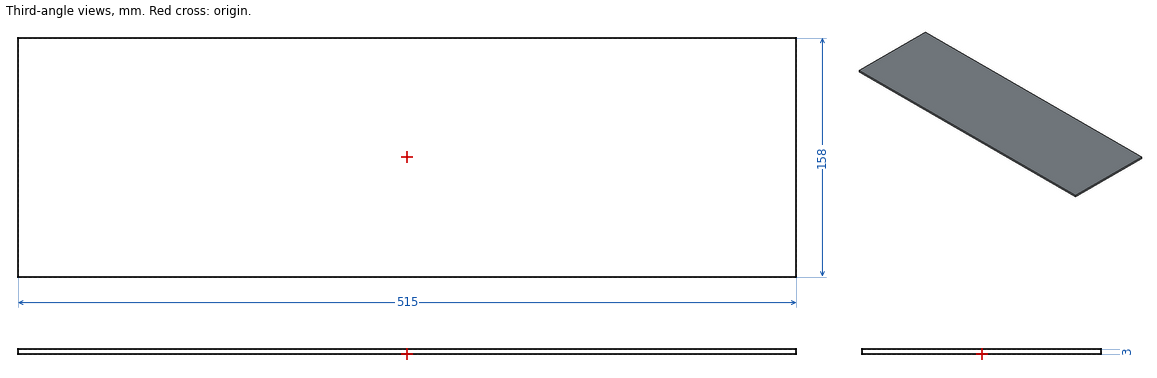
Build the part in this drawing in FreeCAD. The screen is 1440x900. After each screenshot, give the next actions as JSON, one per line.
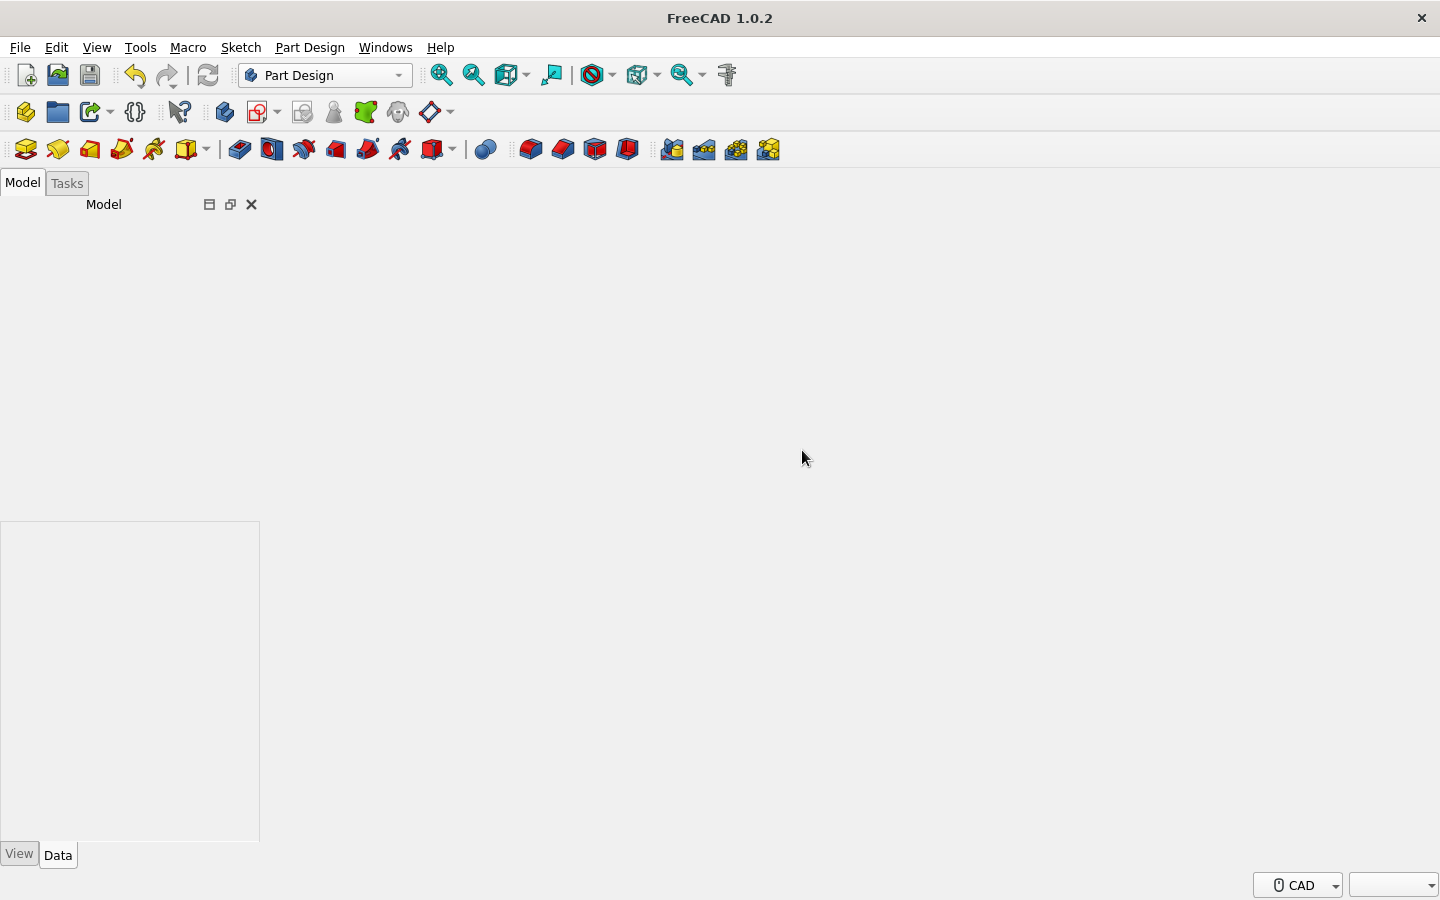
{"action": "left_click", "coordinate": [26, 76]}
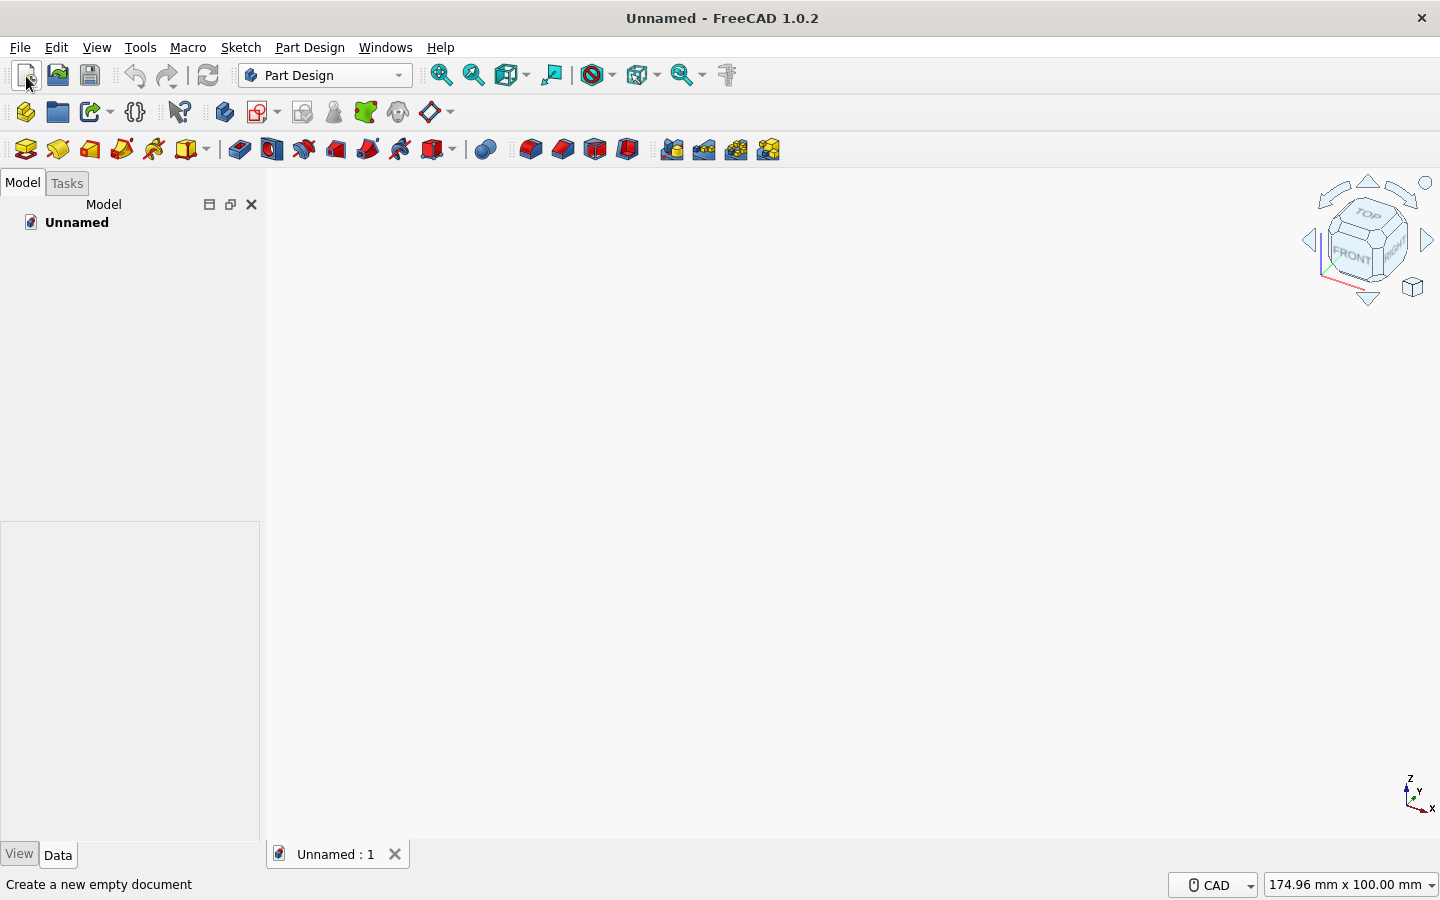
{"action": "left_click", "coordinate": [258, 112]}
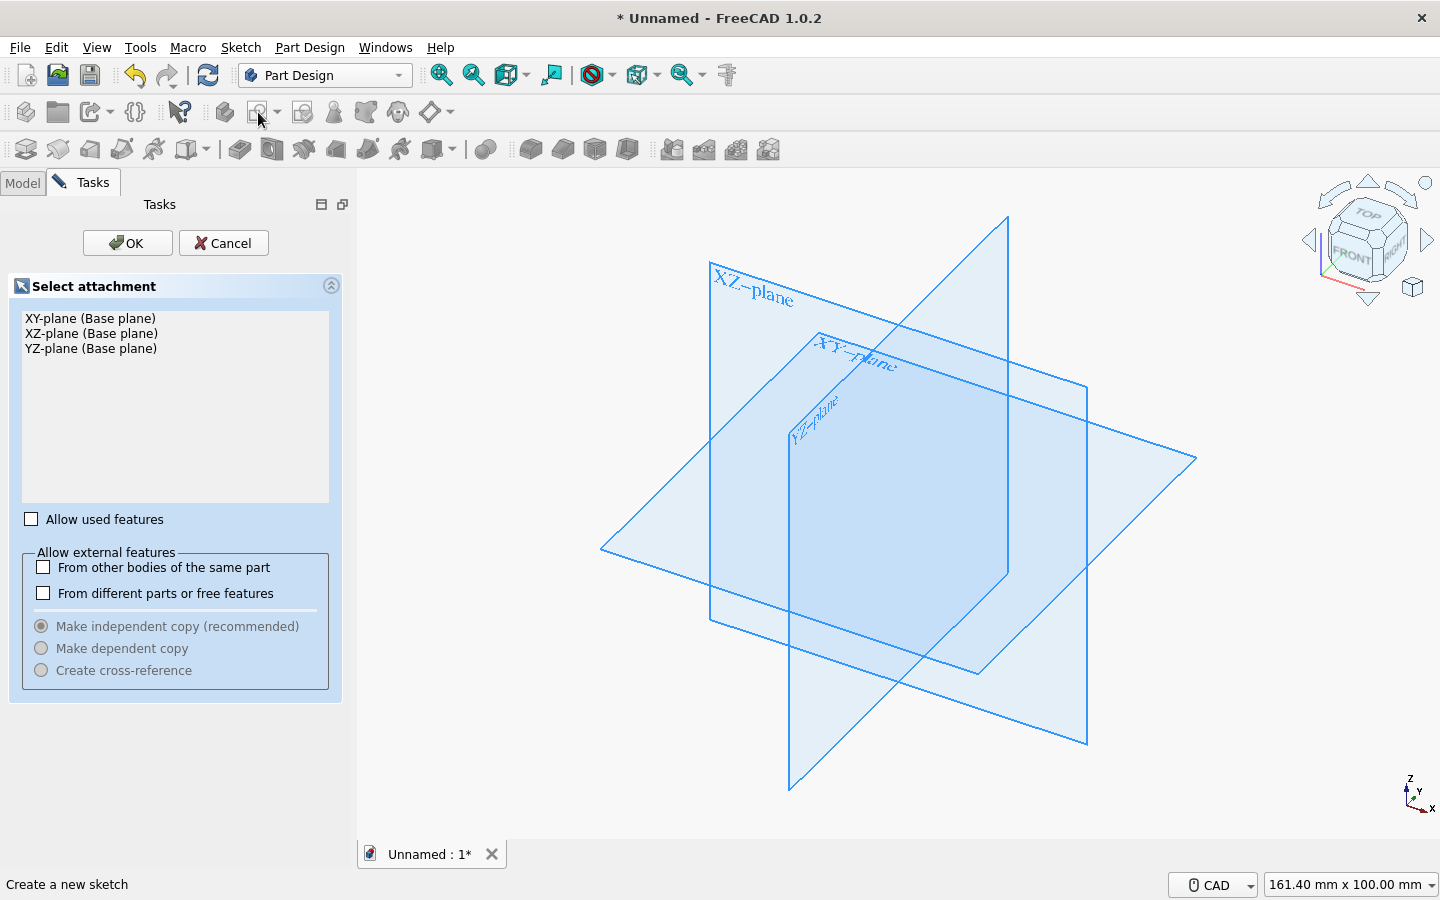
{"action": "left_click", "coordinate": [82, 318]}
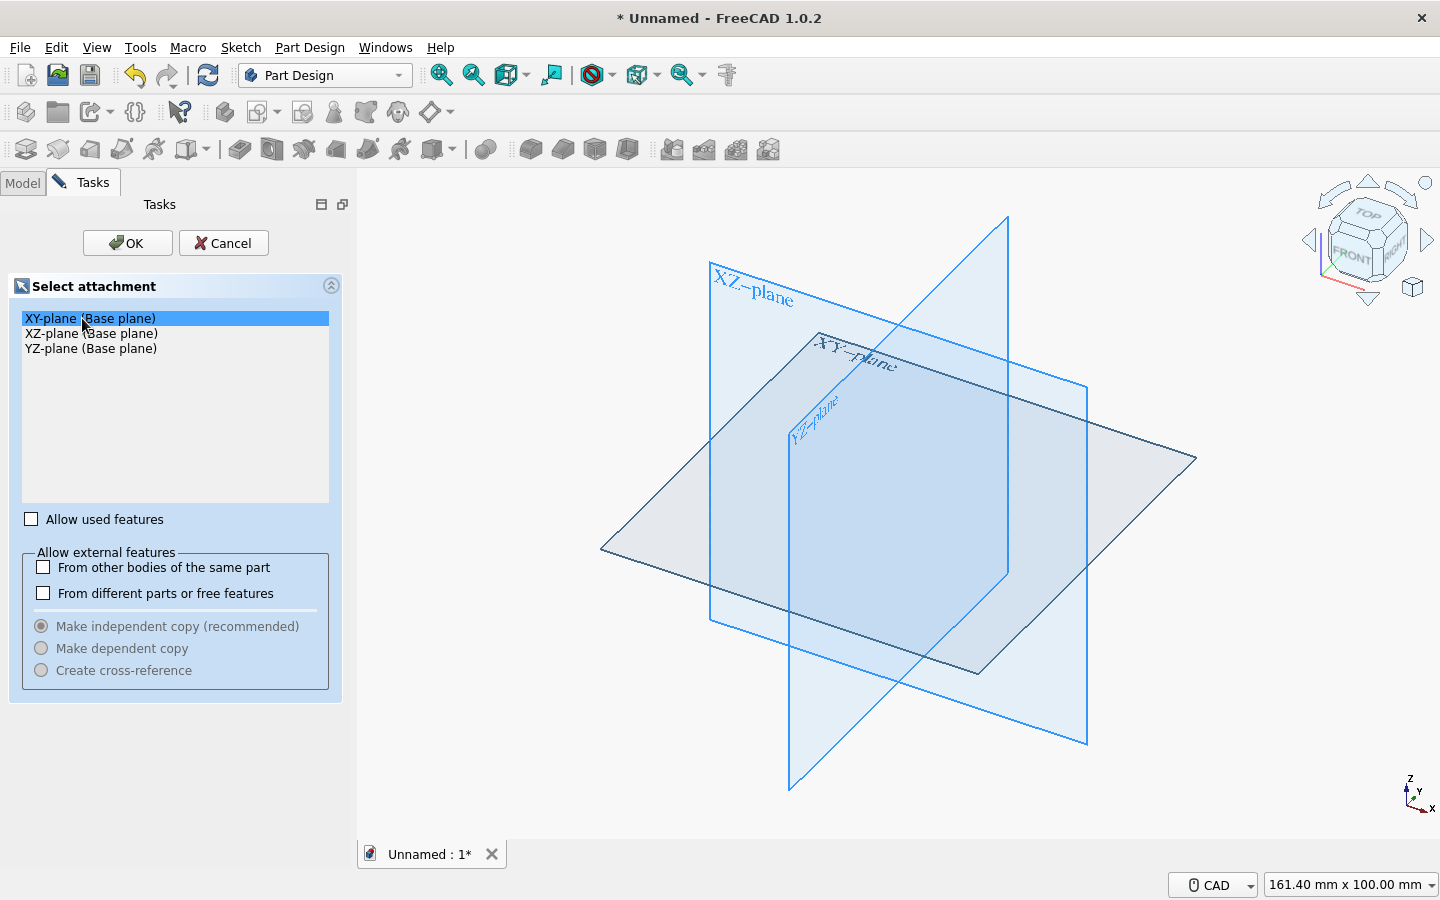
{"action": "left_click", "coordinate": [128, 243]}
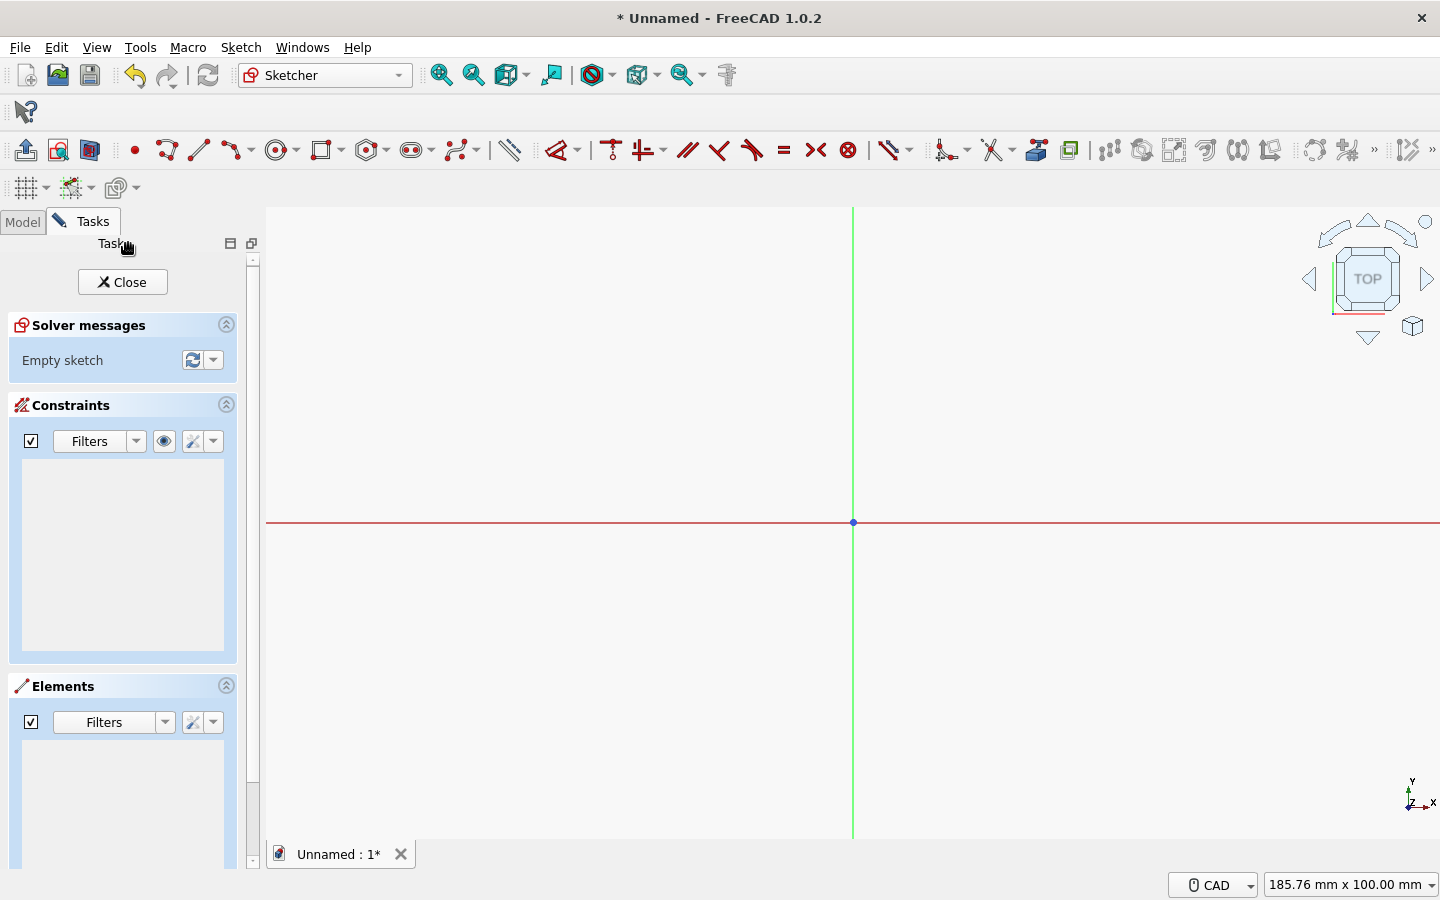
{"action": "scroll", "coordinate": [767, 523], "scroll_direction": "down", "scroll_amount": 8}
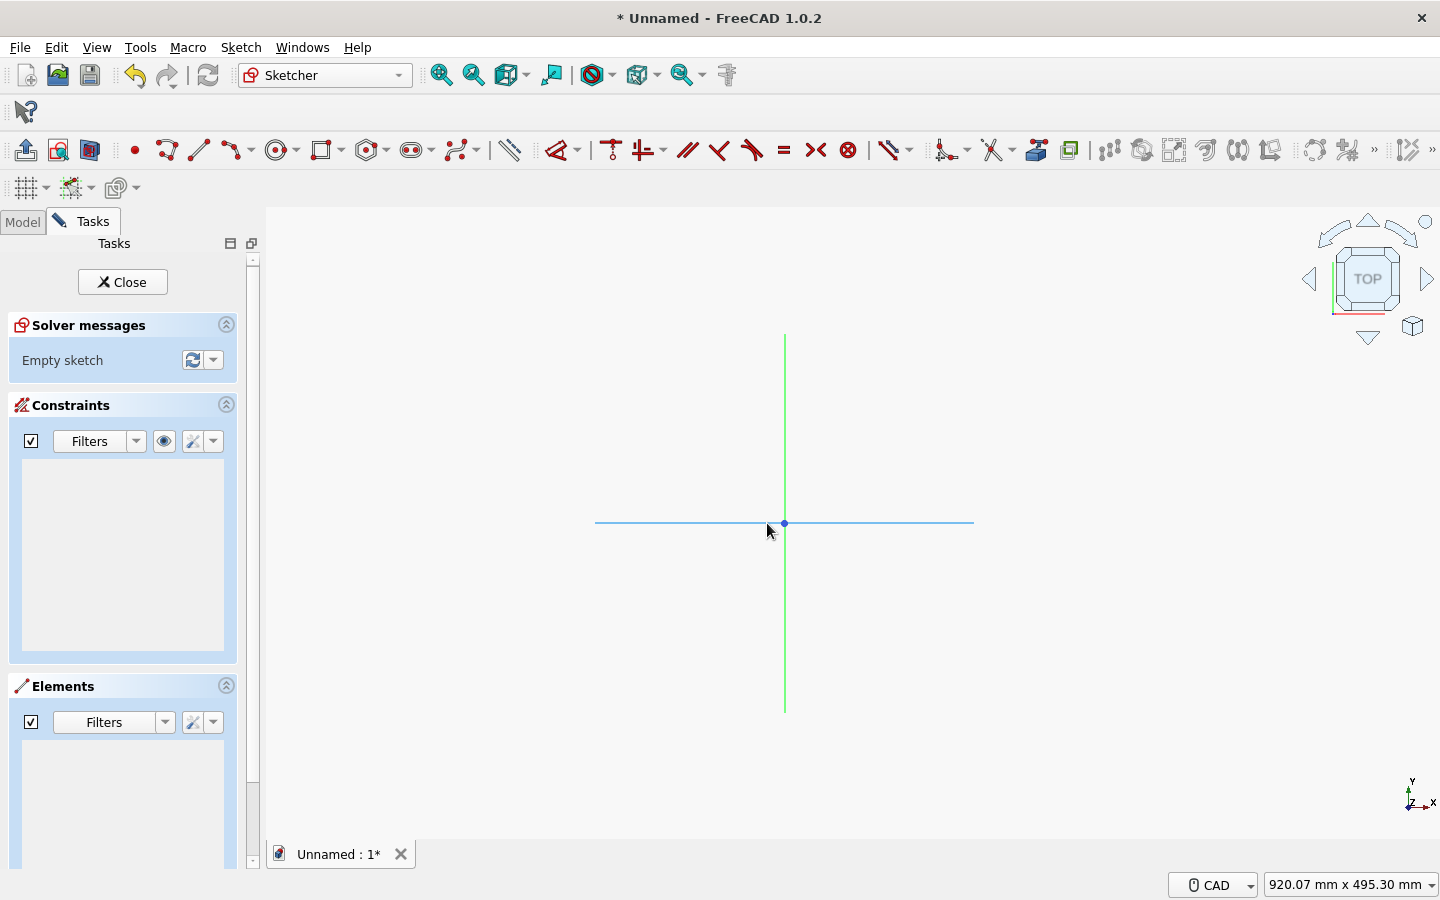
{"action": "left_click", "coordinate": [344, 150]}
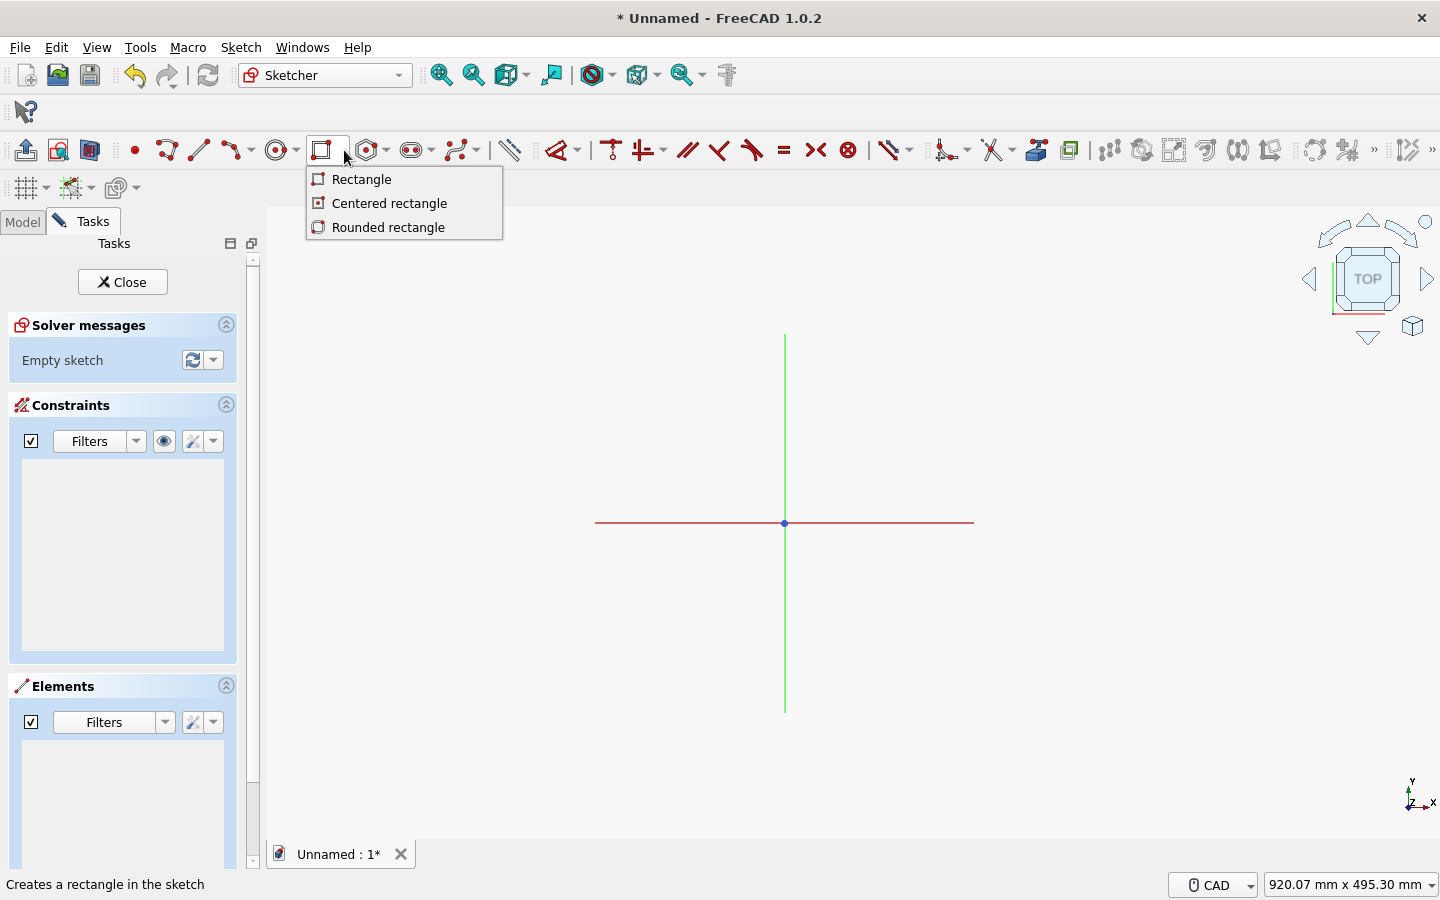
{"action": "left_click", "coordinate": [404, 203]}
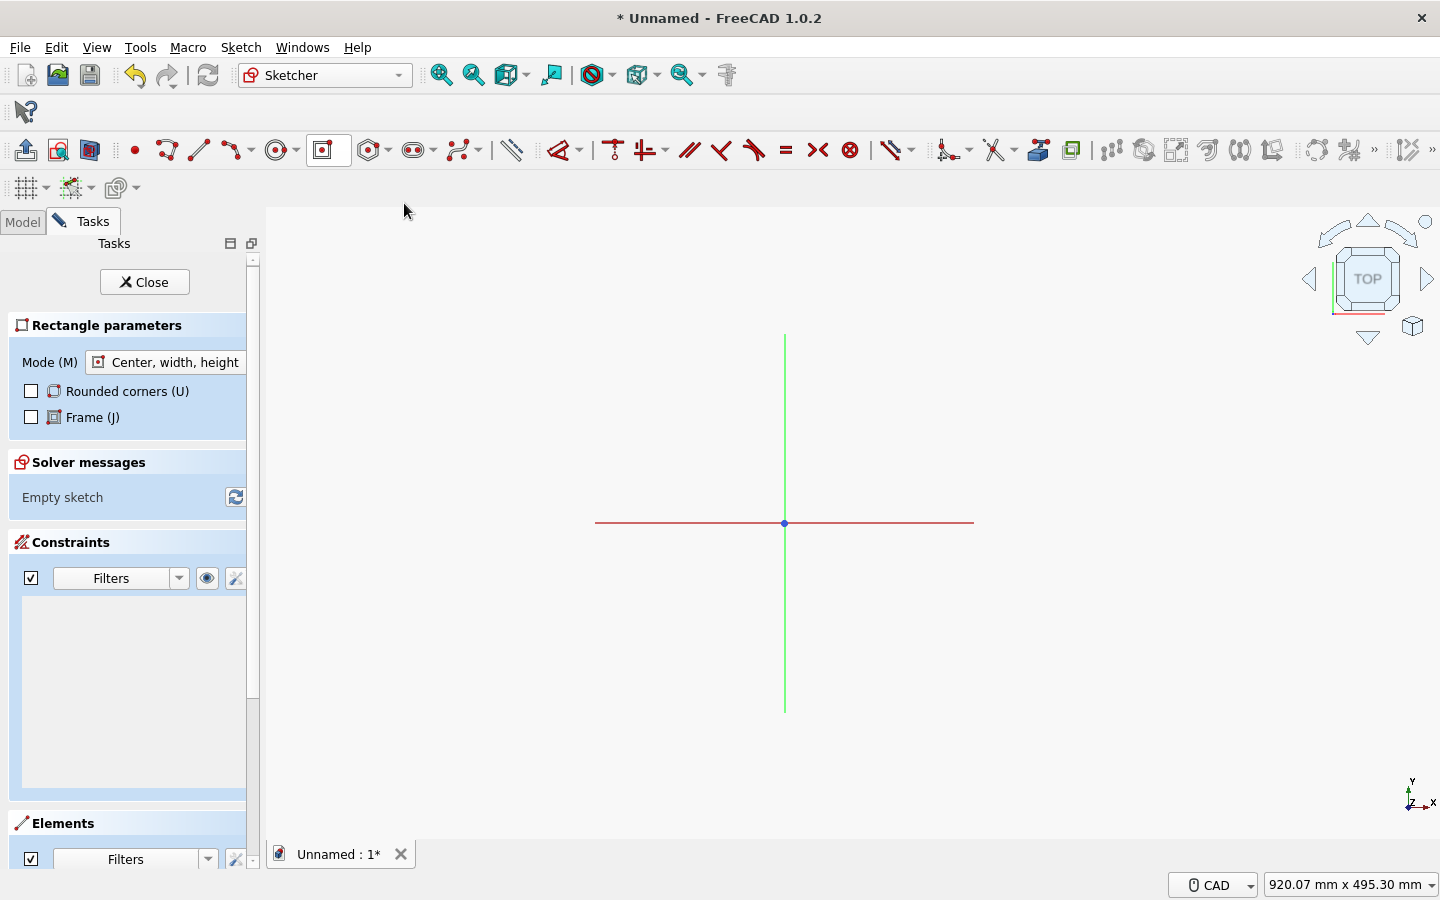
{"action": "left_click", "coordinate": [785, 523]}
{"action": "mouse_move", "coordinate": [1113, 423]}